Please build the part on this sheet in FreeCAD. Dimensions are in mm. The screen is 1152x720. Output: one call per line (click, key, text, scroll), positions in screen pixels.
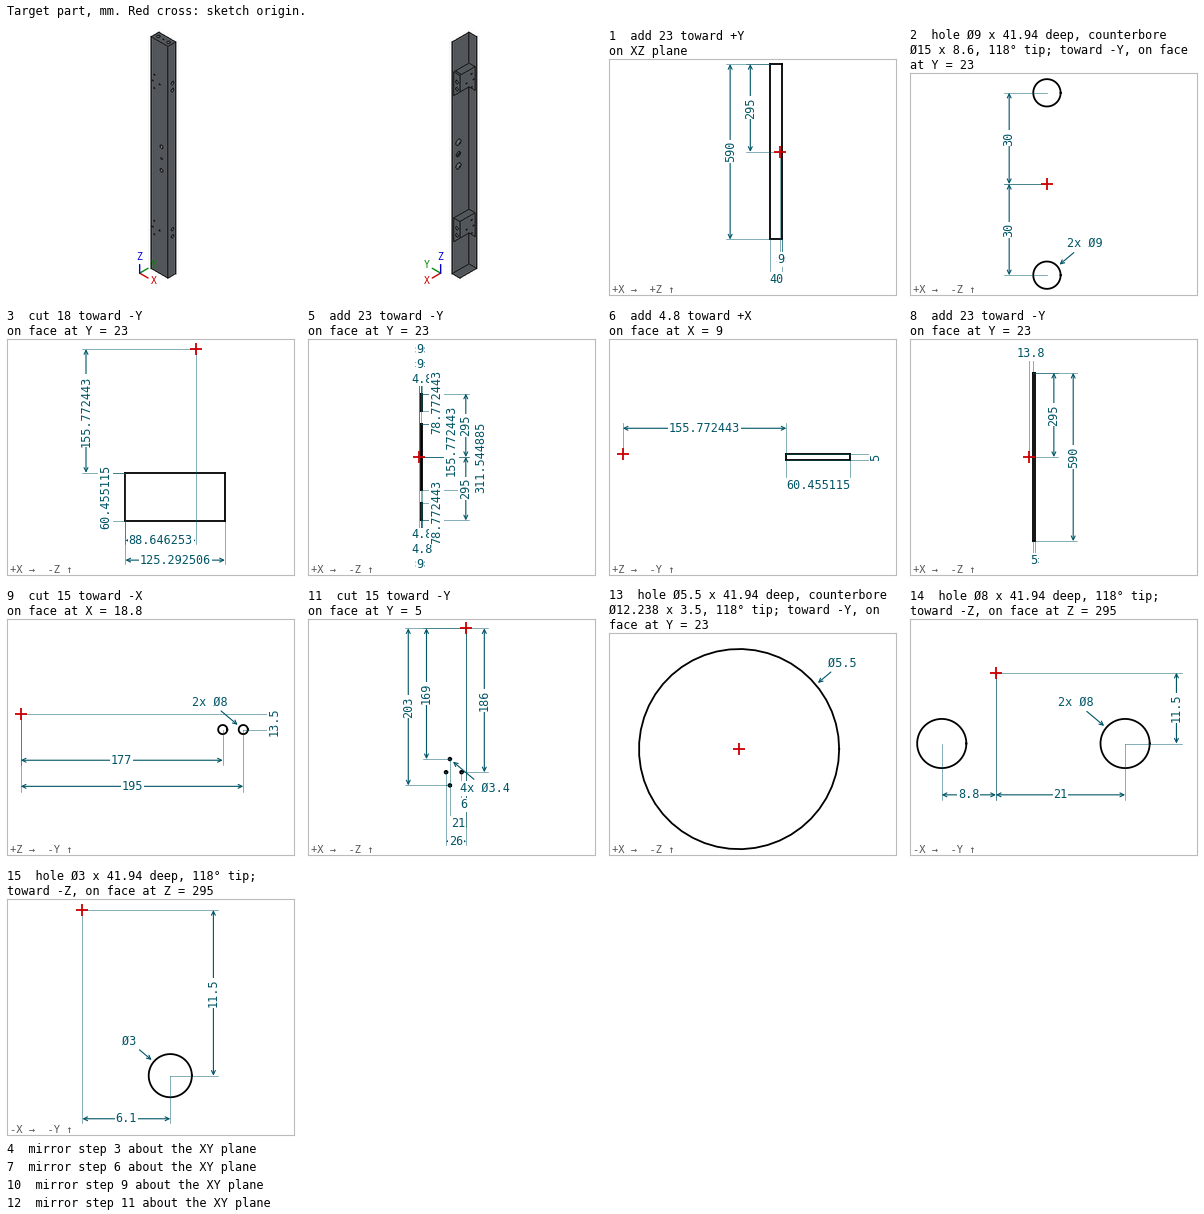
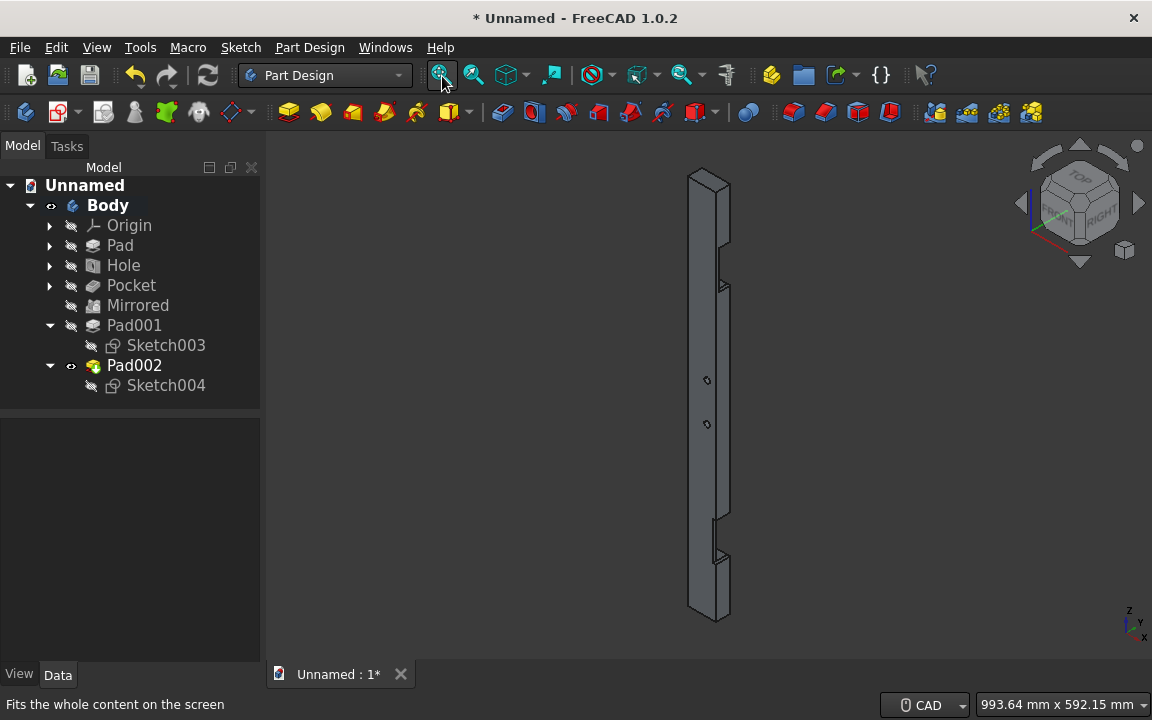
click(116, 366)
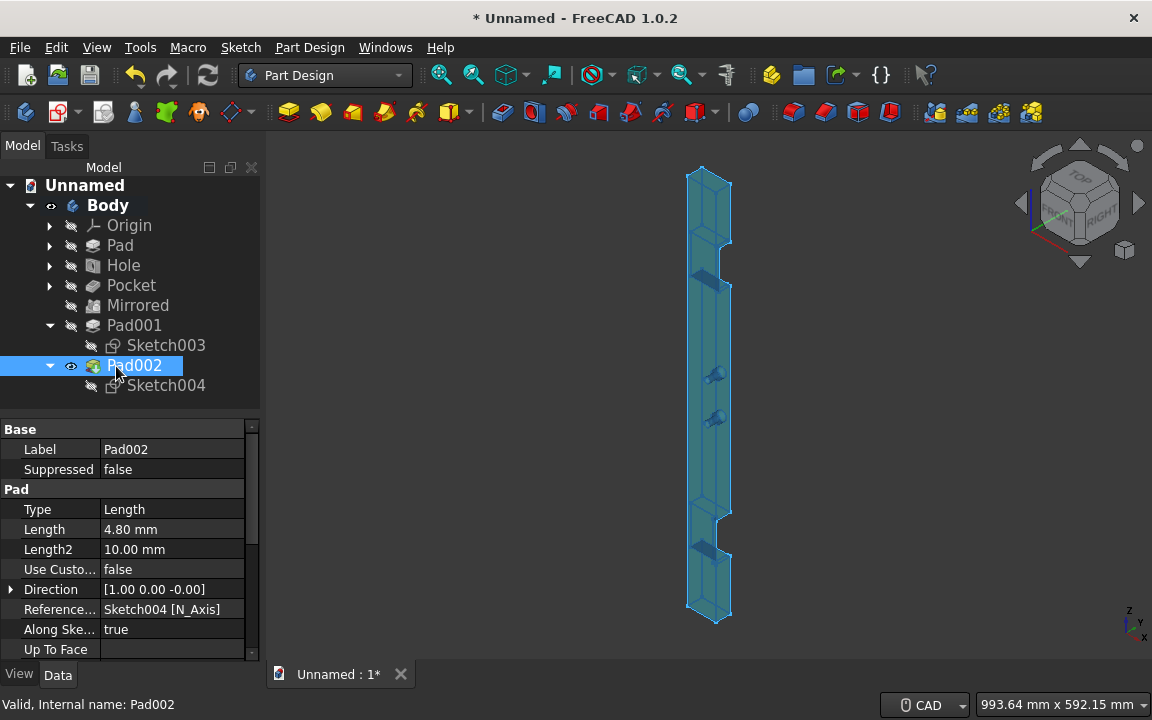
click(936, 112)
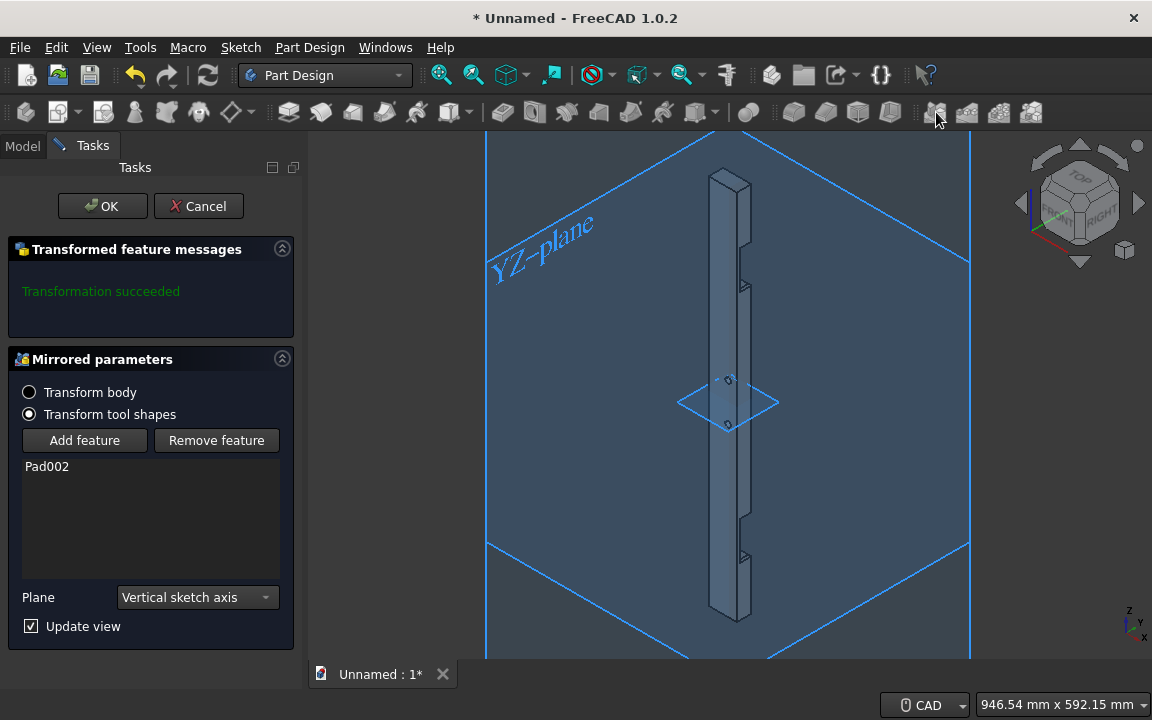
click(198, 598)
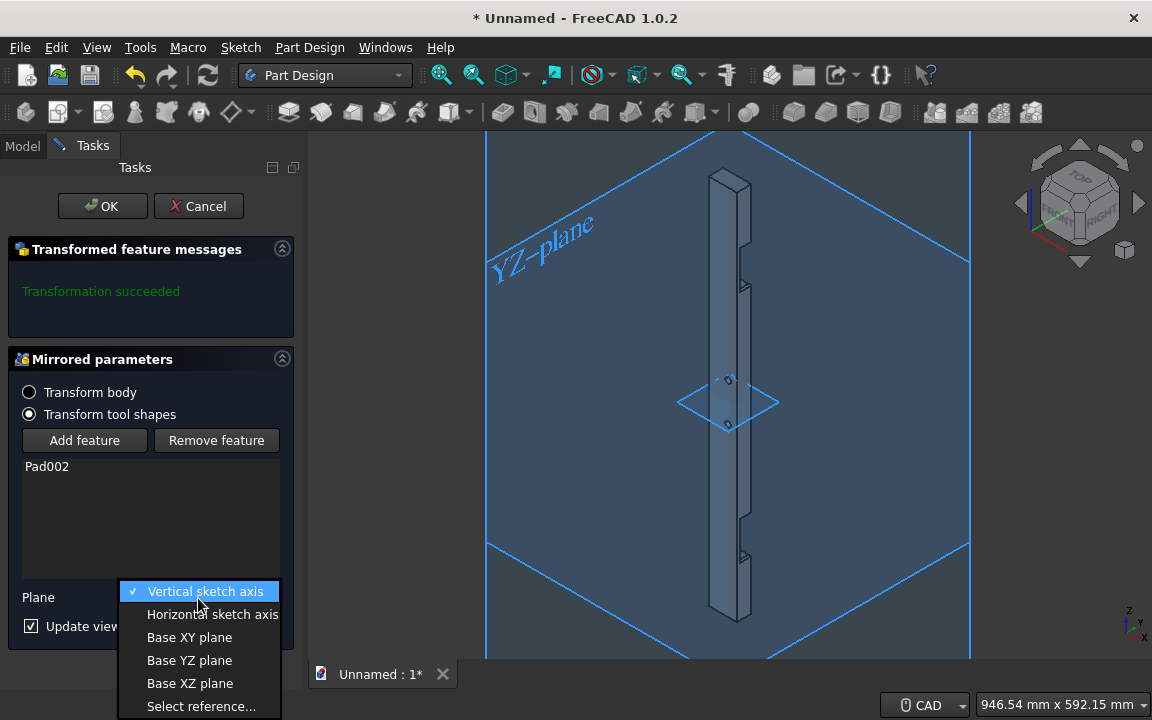
click(198, 638)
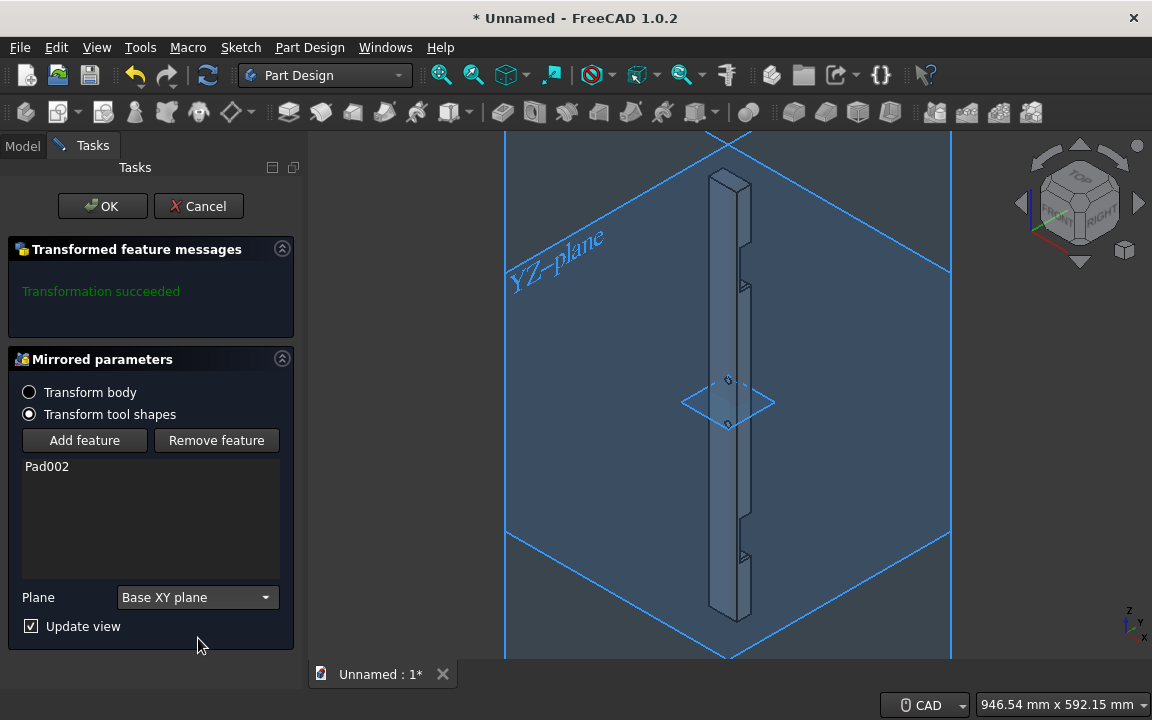
click(103, 206)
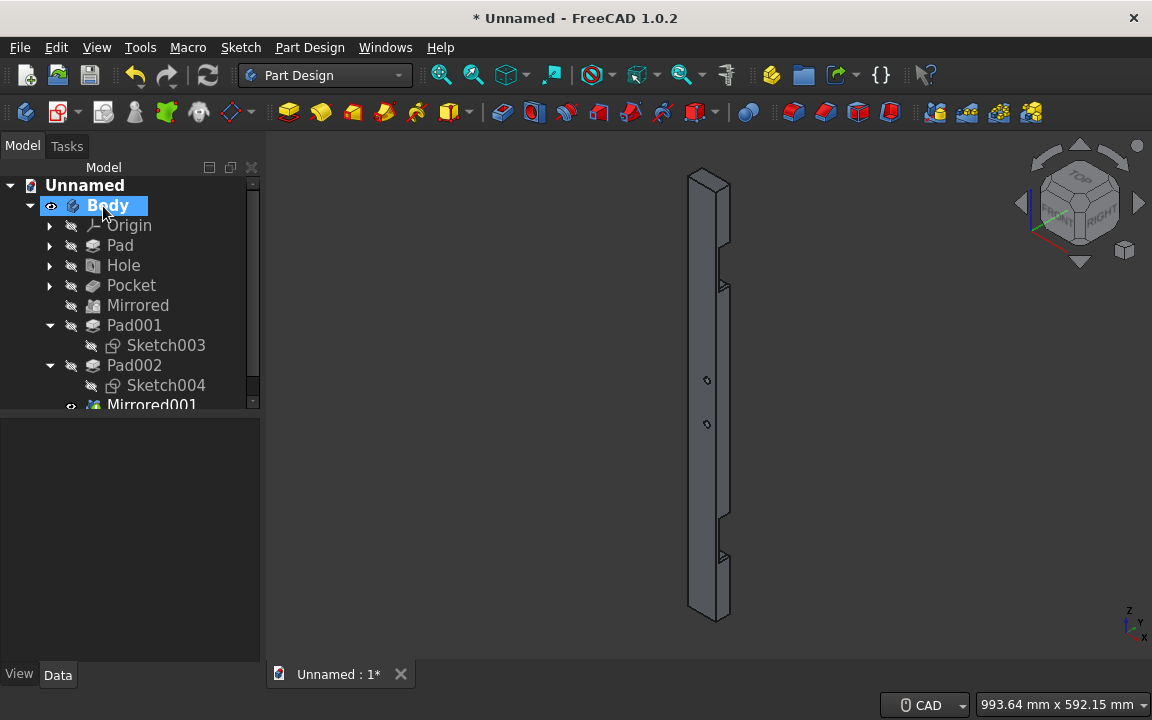
key(4)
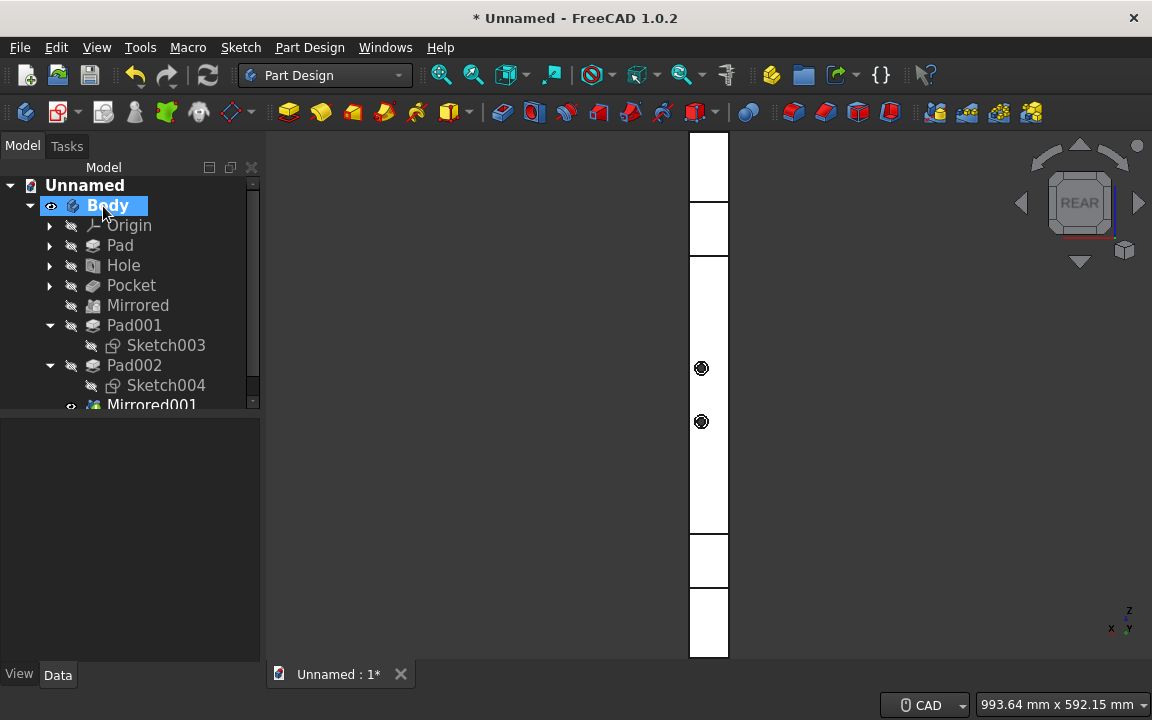
click(709, 473)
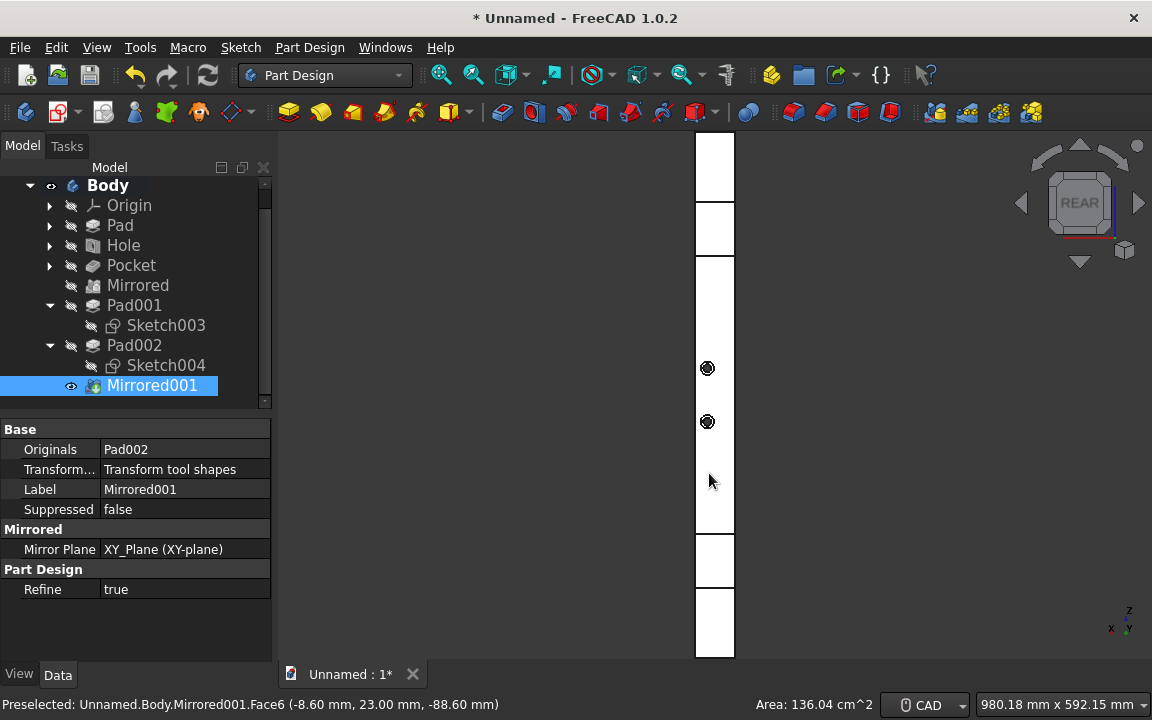
click(58, 112)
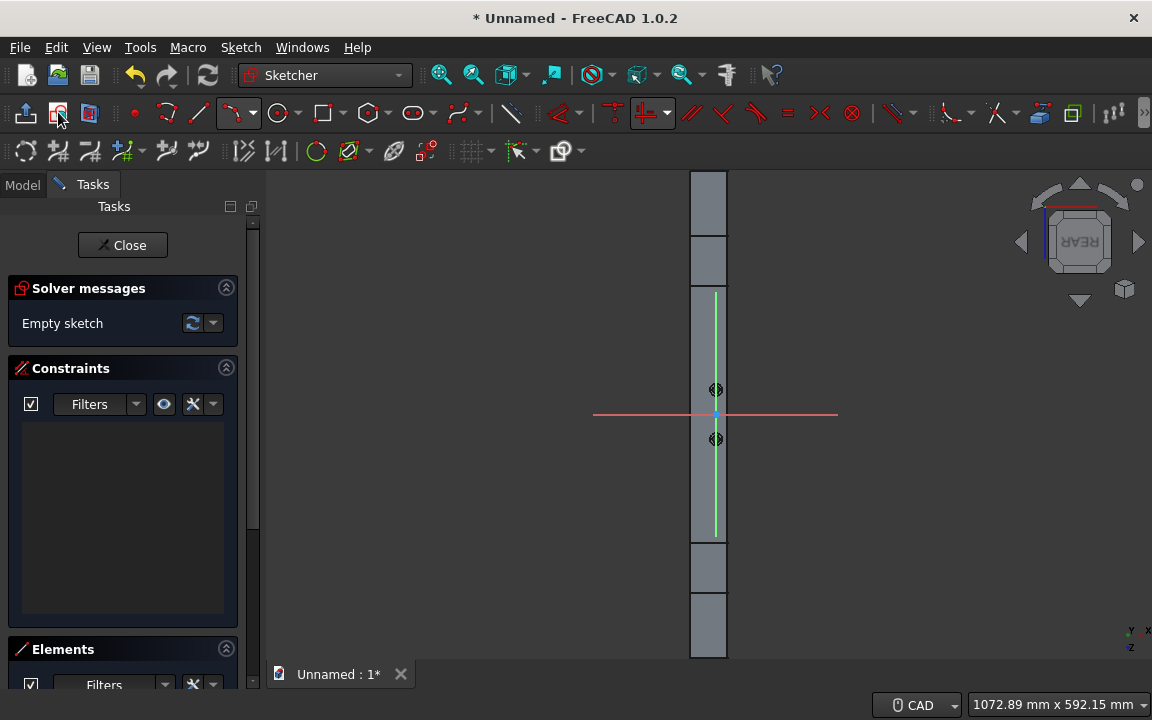
scroll(471, 414, down, 2)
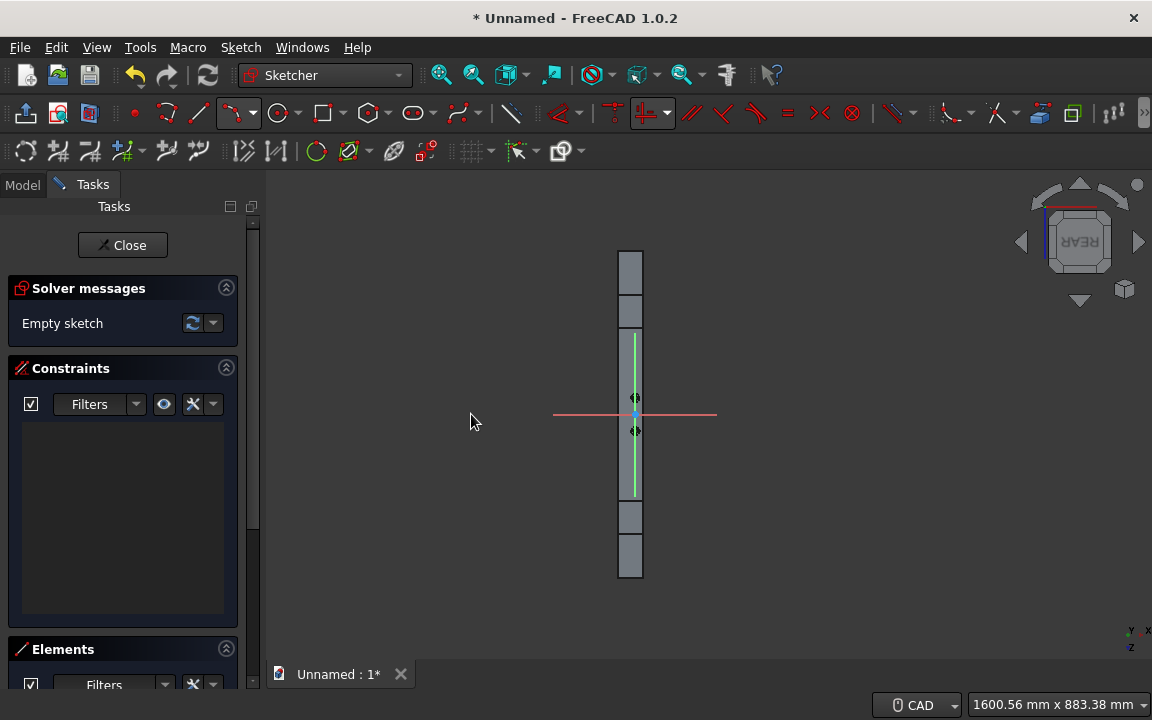
click(324, 114)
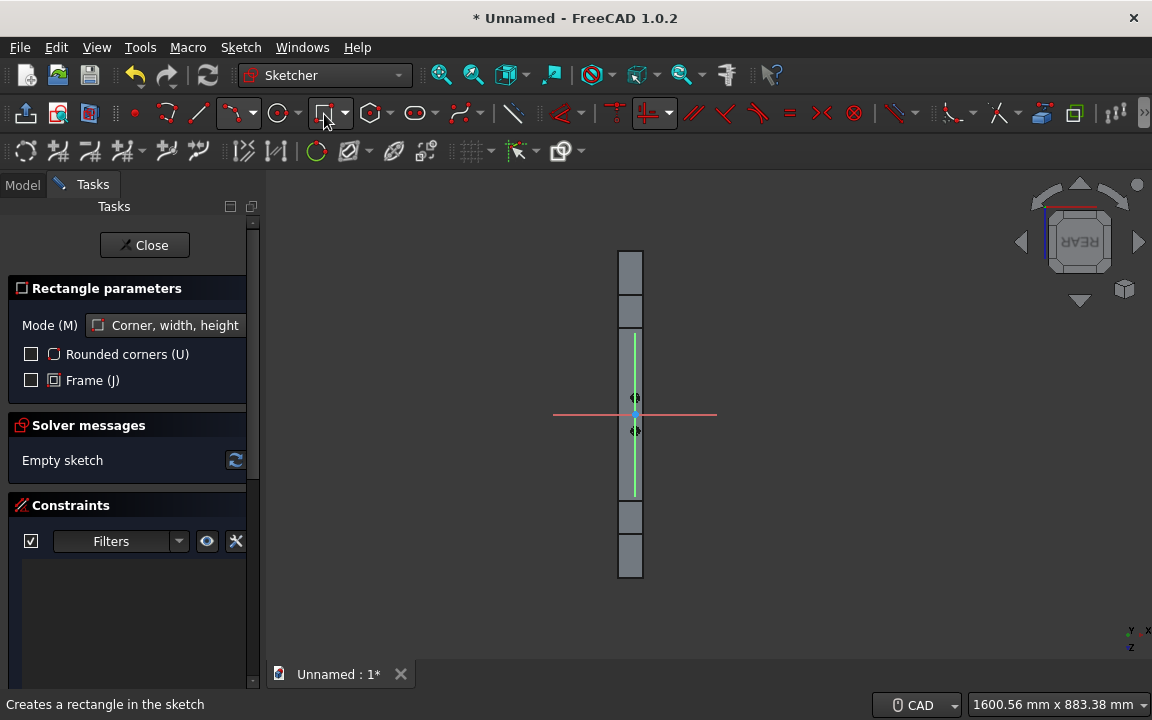
scroll(643, 251, up, 9)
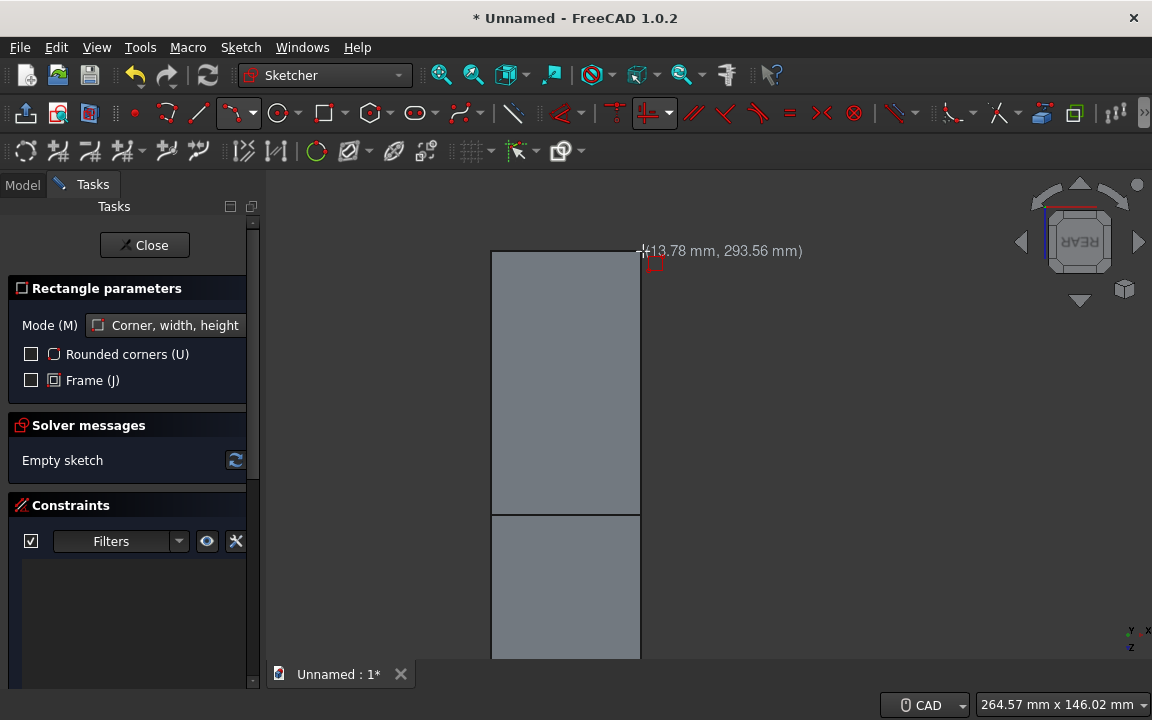
scroll(643, 251, down, 9)